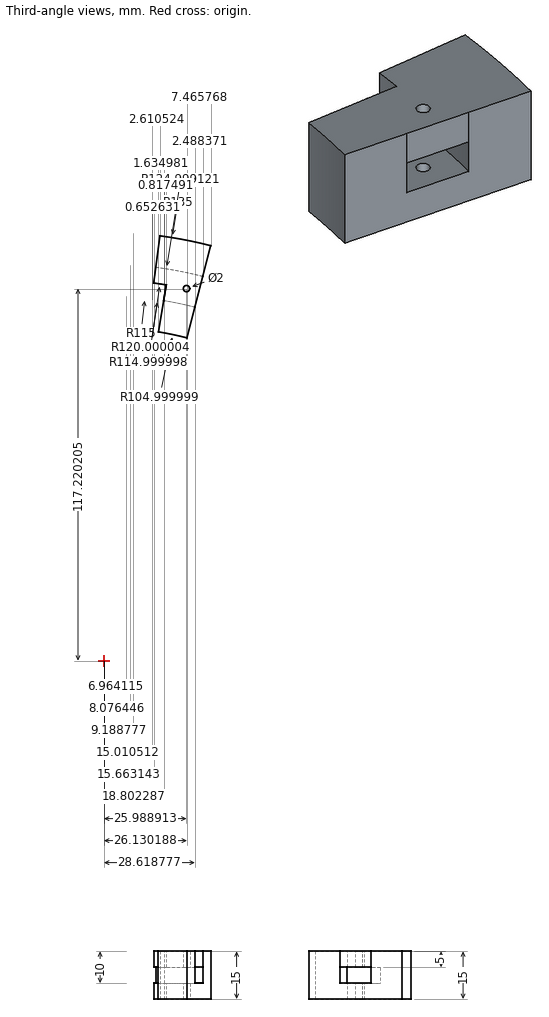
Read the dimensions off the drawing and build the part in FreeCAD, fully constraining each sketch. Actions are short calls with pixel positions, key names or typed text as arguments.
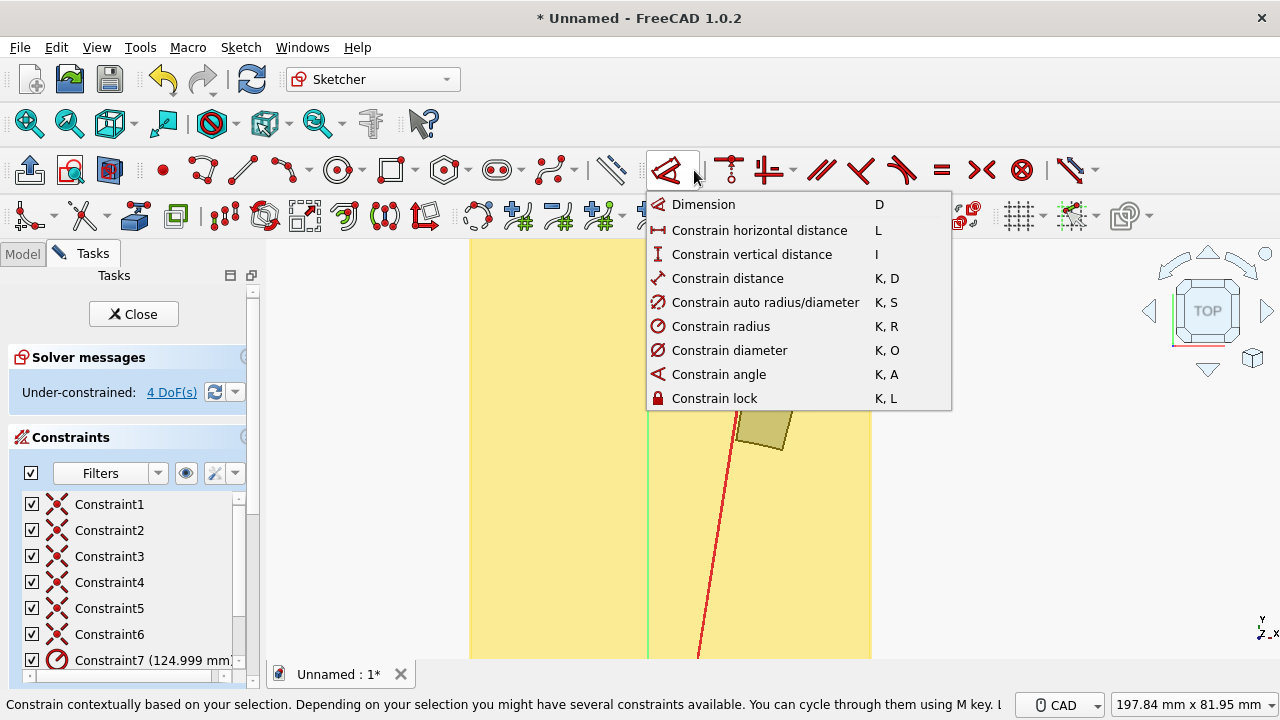
click(799, 230)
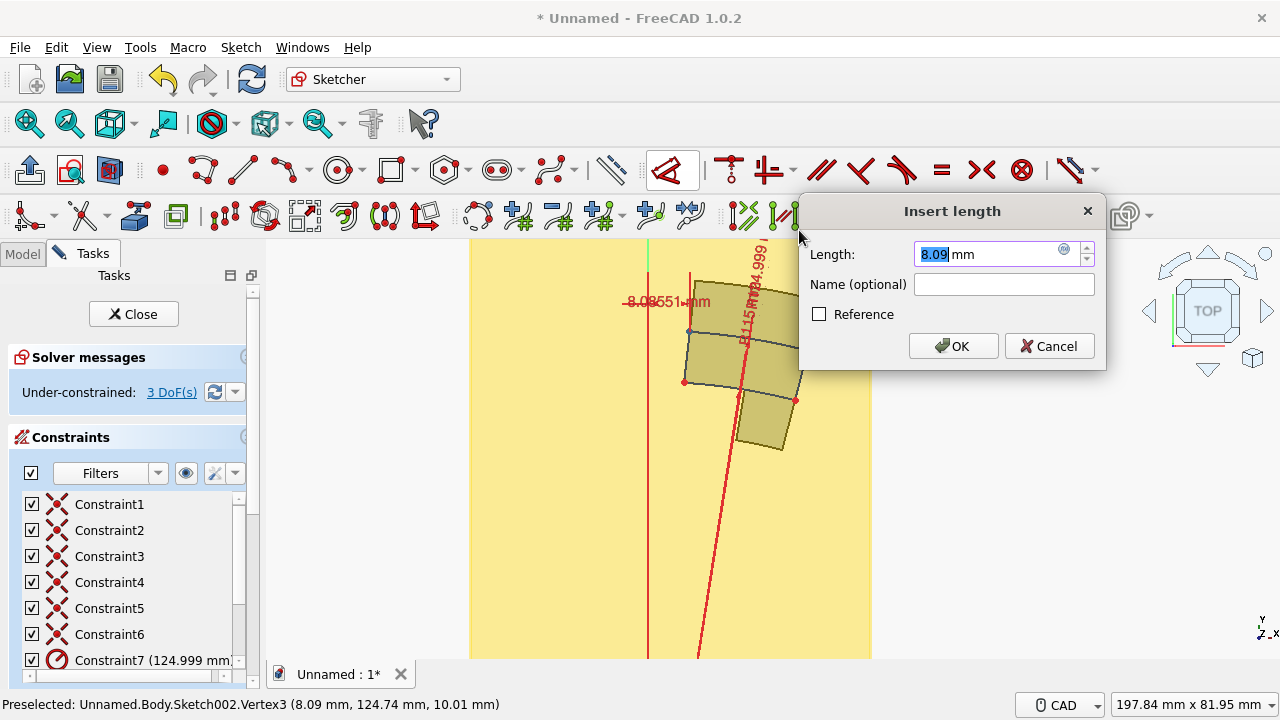
text(8.076446)
key(Return)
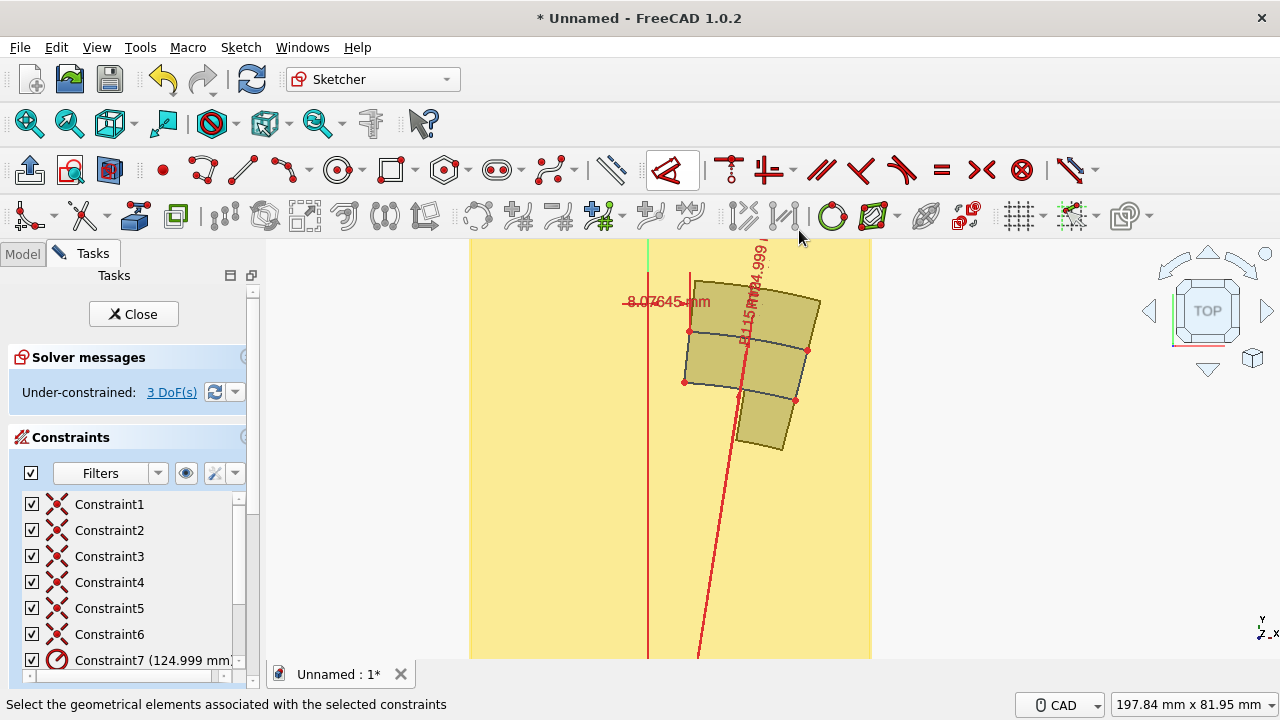
click(684, 383)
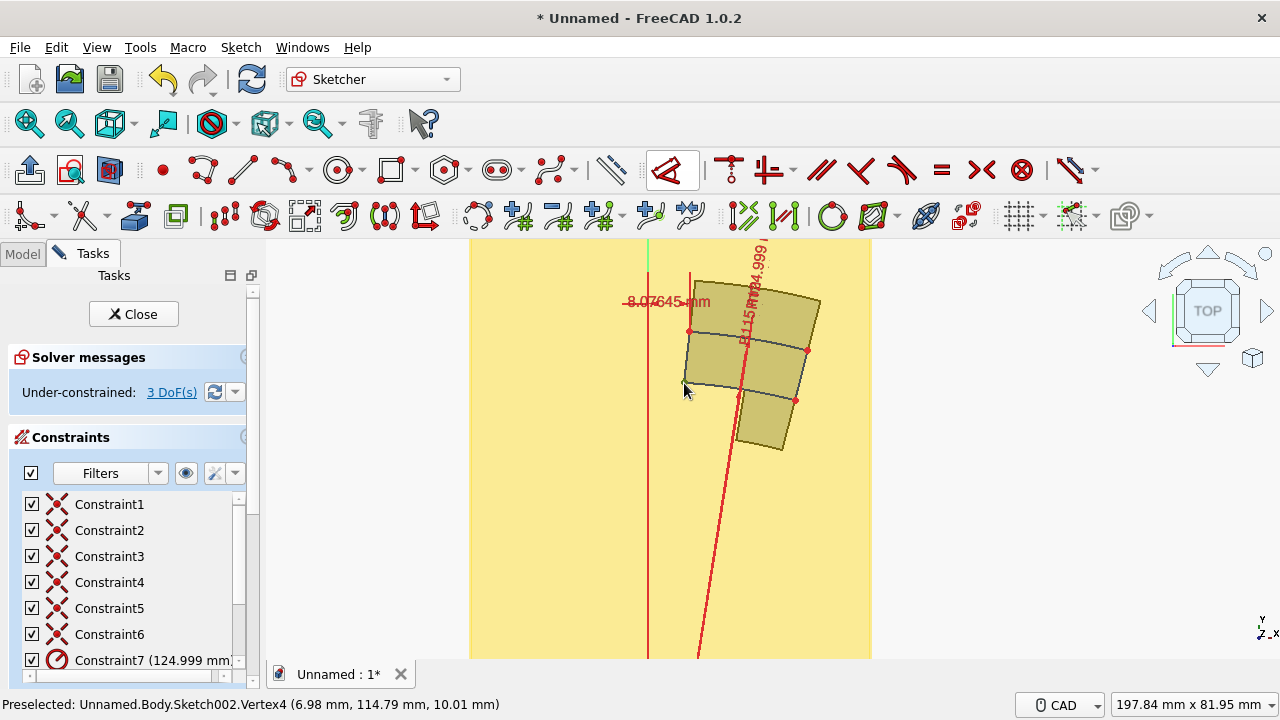
click(694, 170)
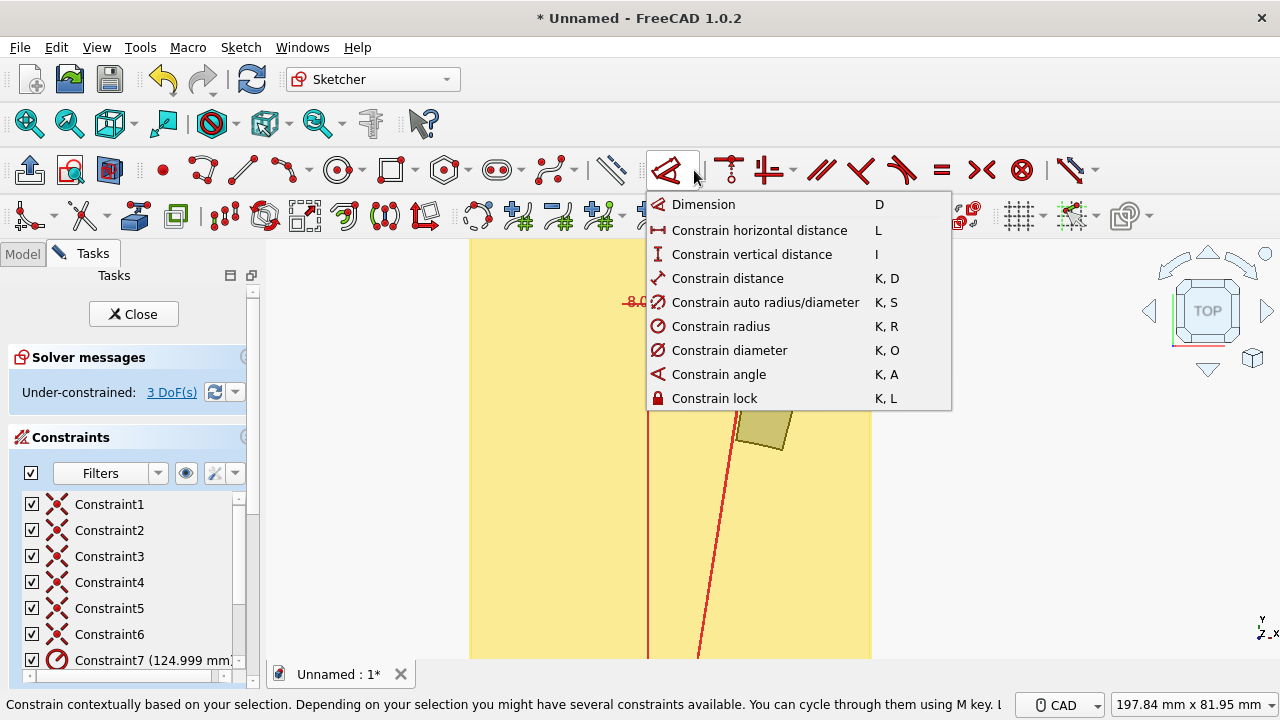
click(799, 230)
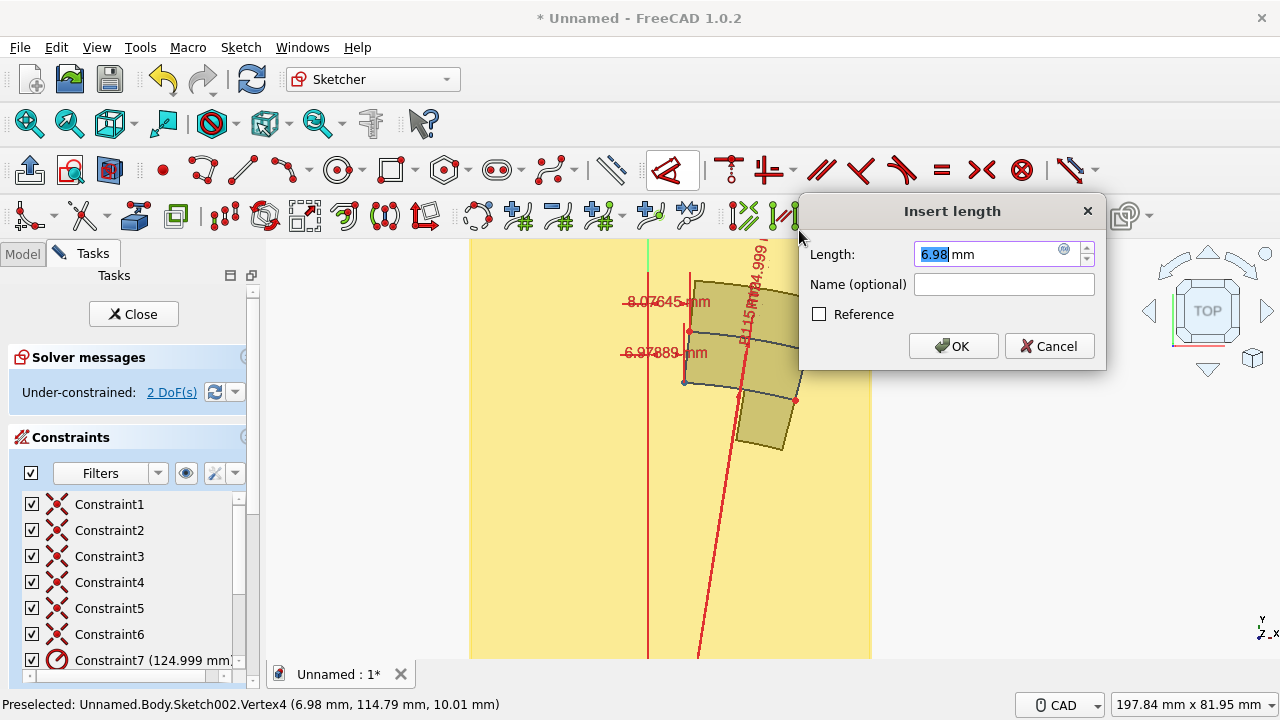
text(6.964115)
key(Return)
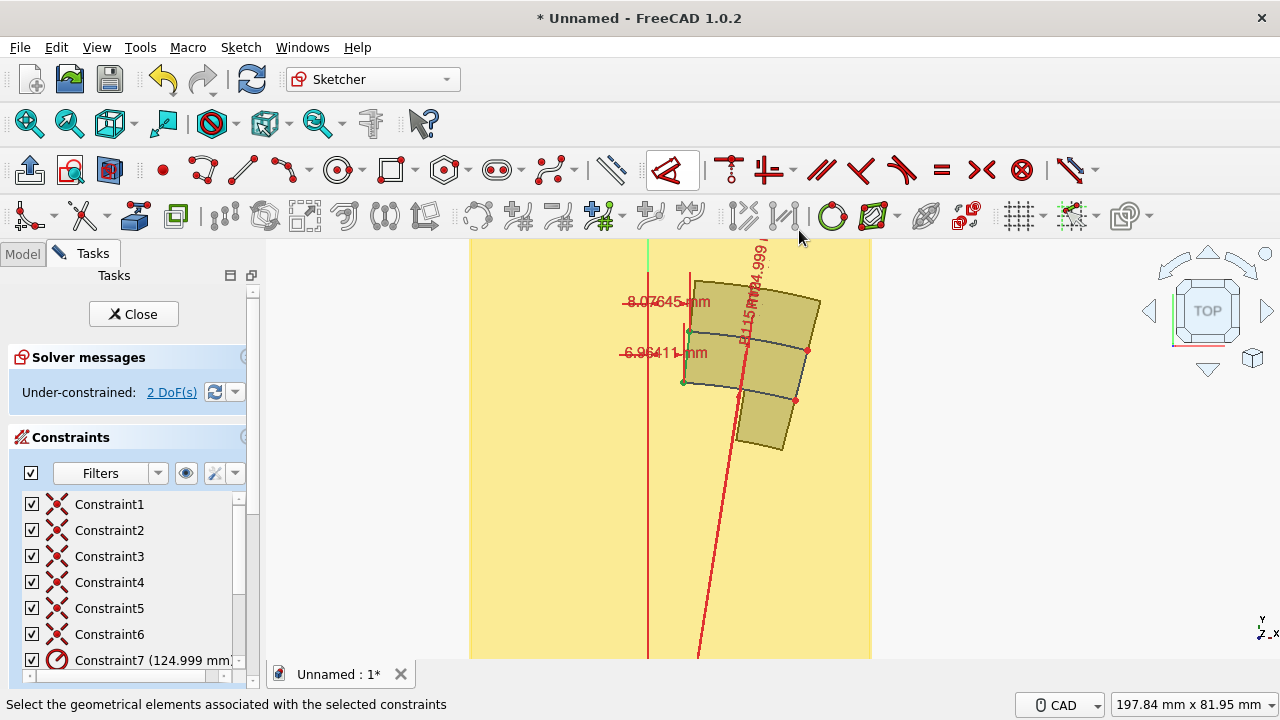
scroll(799, 385, up, 6)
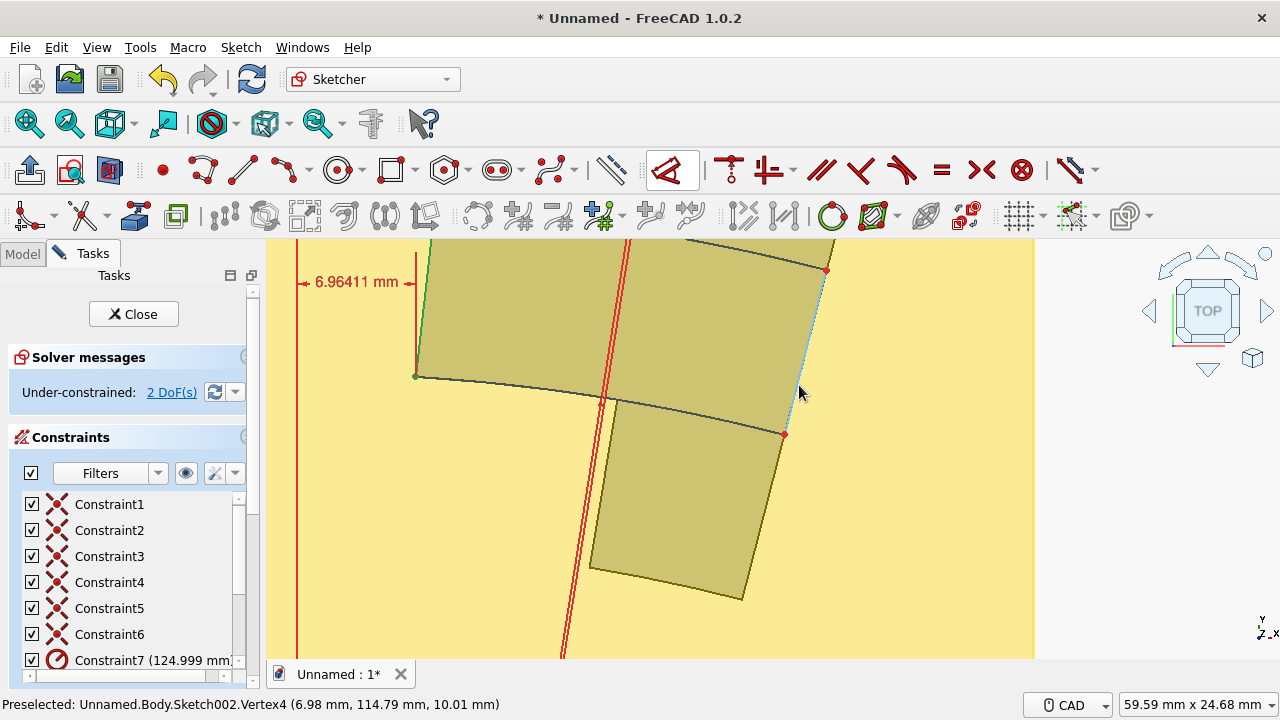
click(797, 385)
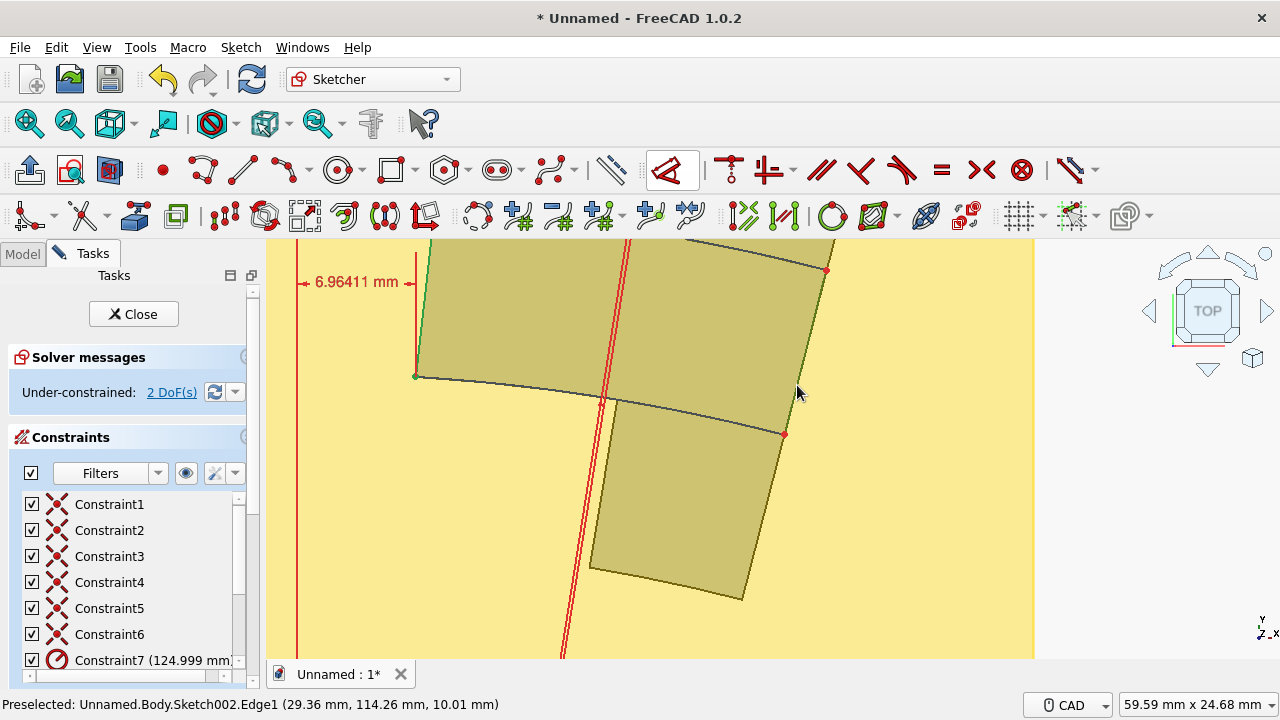
click(694, 170)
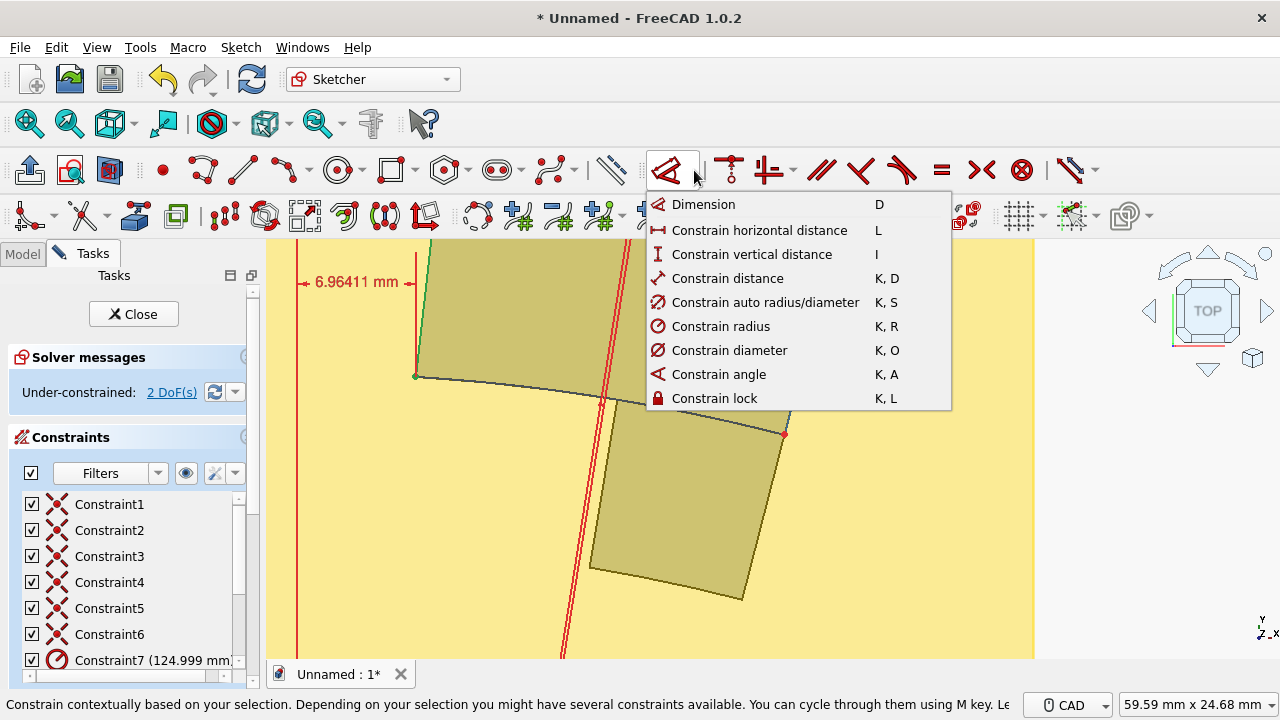
click(799, 230)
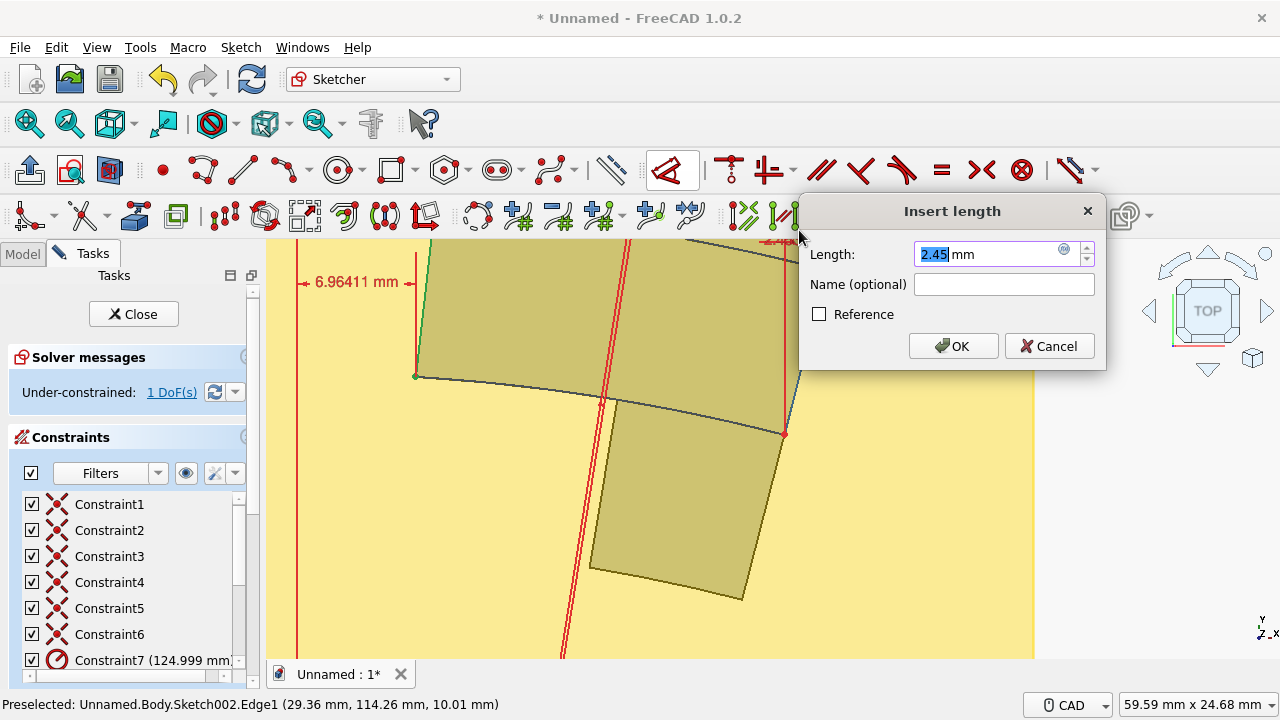
text(2.488371)
key(Return)